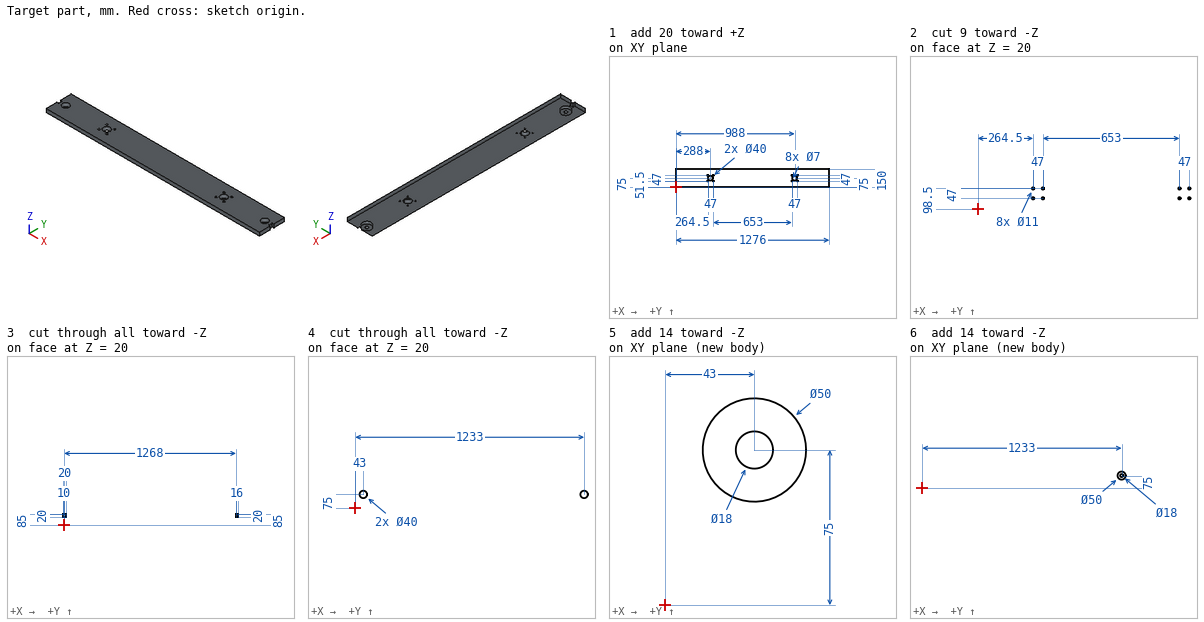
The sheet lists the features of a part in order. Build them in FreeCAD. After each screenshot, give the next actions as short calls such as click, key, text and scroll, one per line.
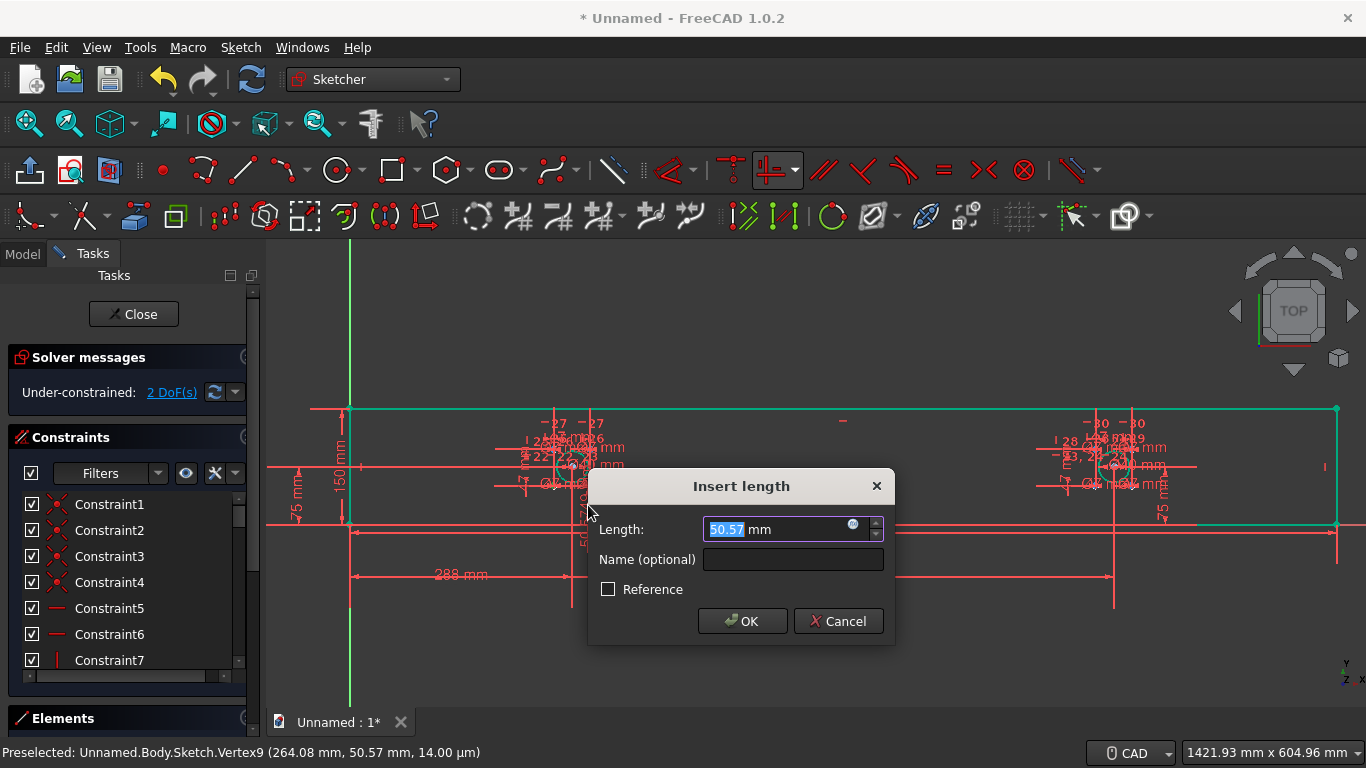
text(51.5)
key(Return)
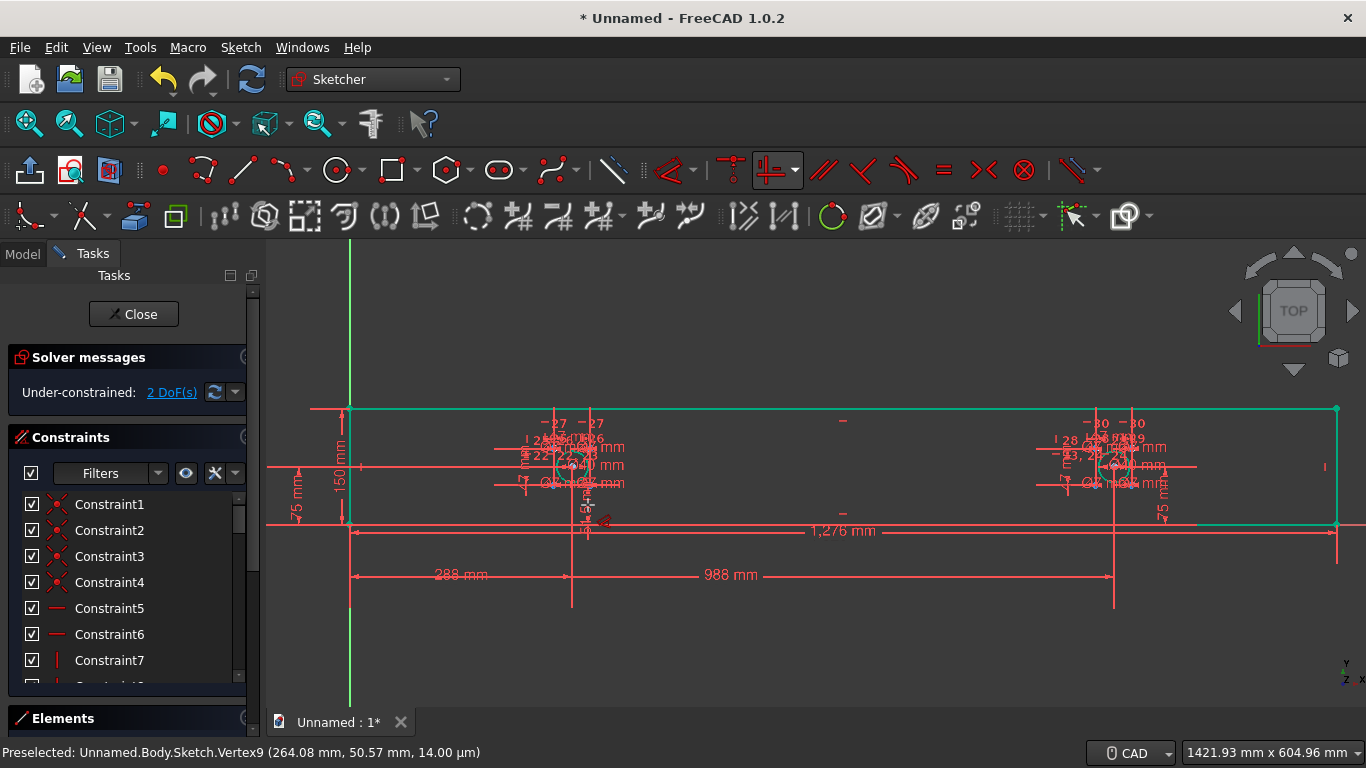
click(590, 485)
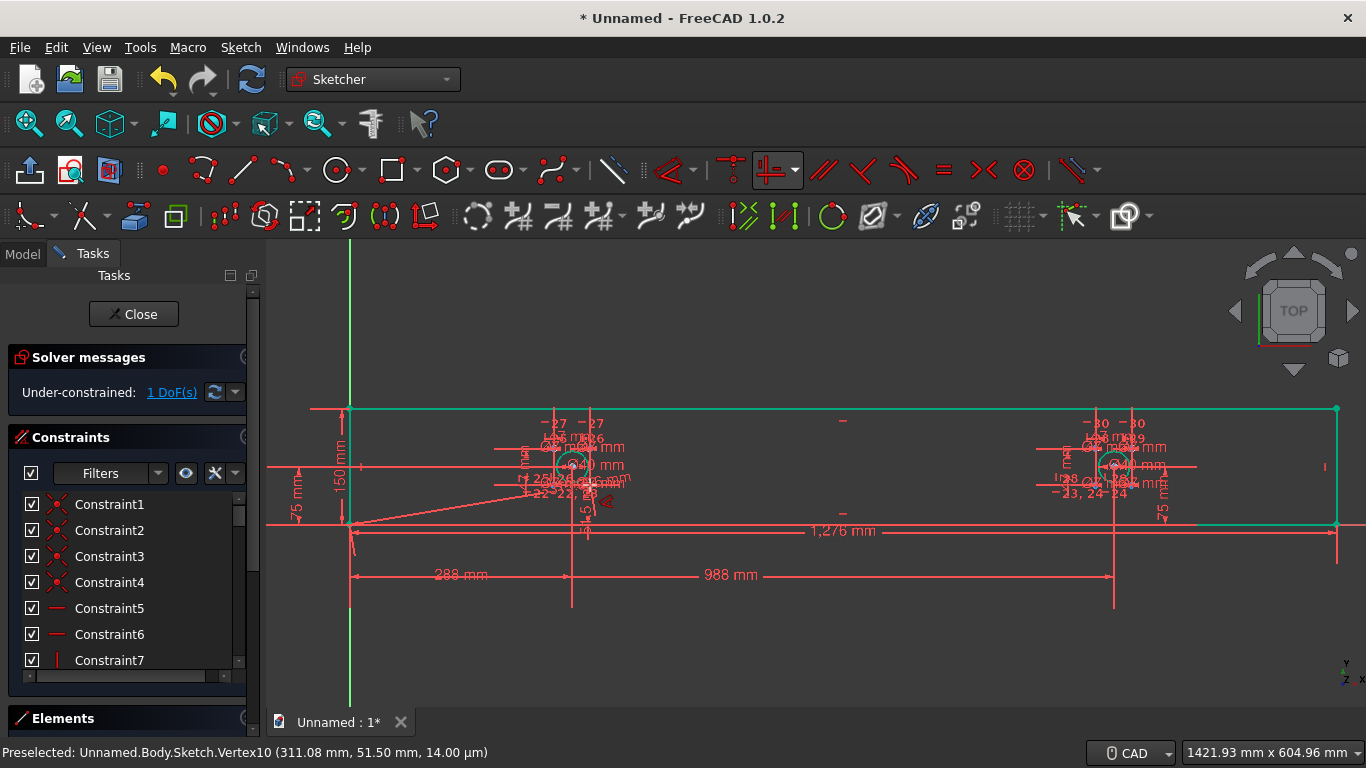
click(1096, 485)
click(843, 451)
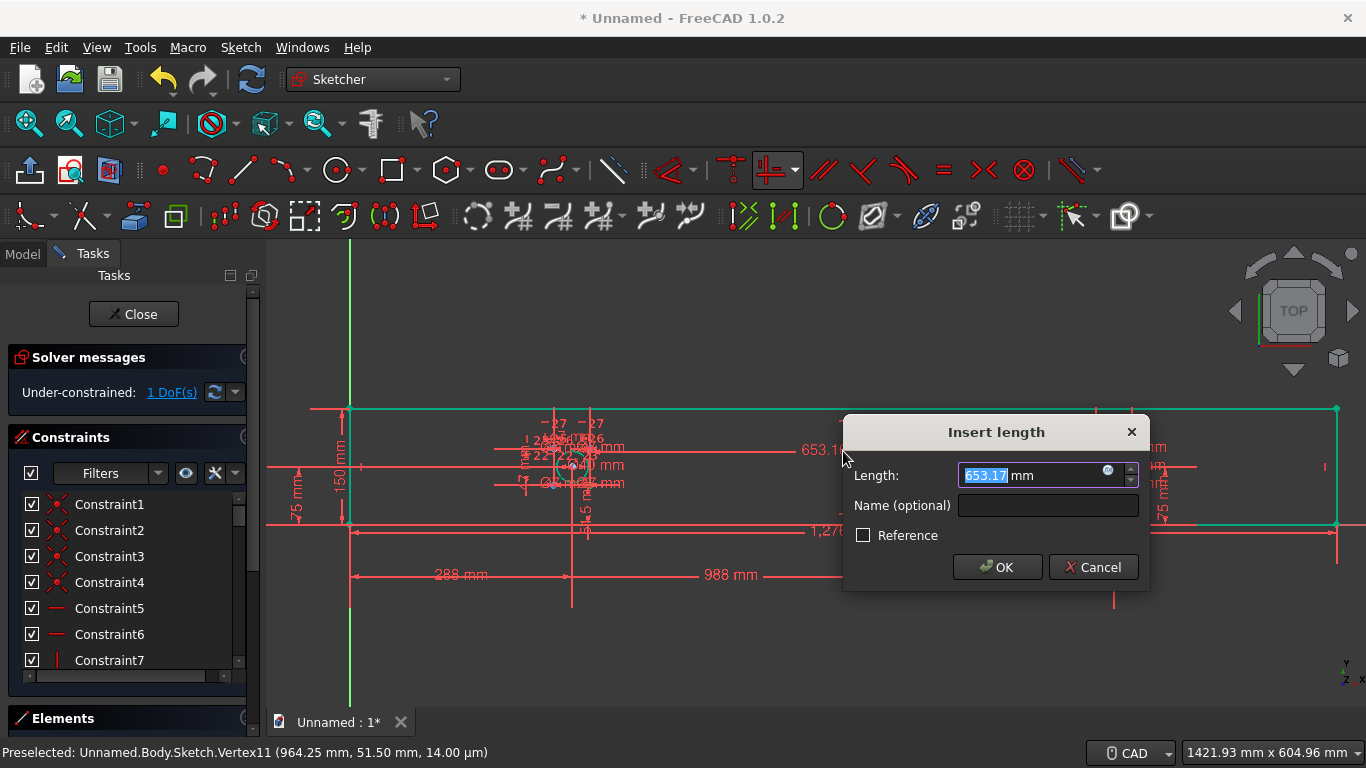
text(653)
key(Return)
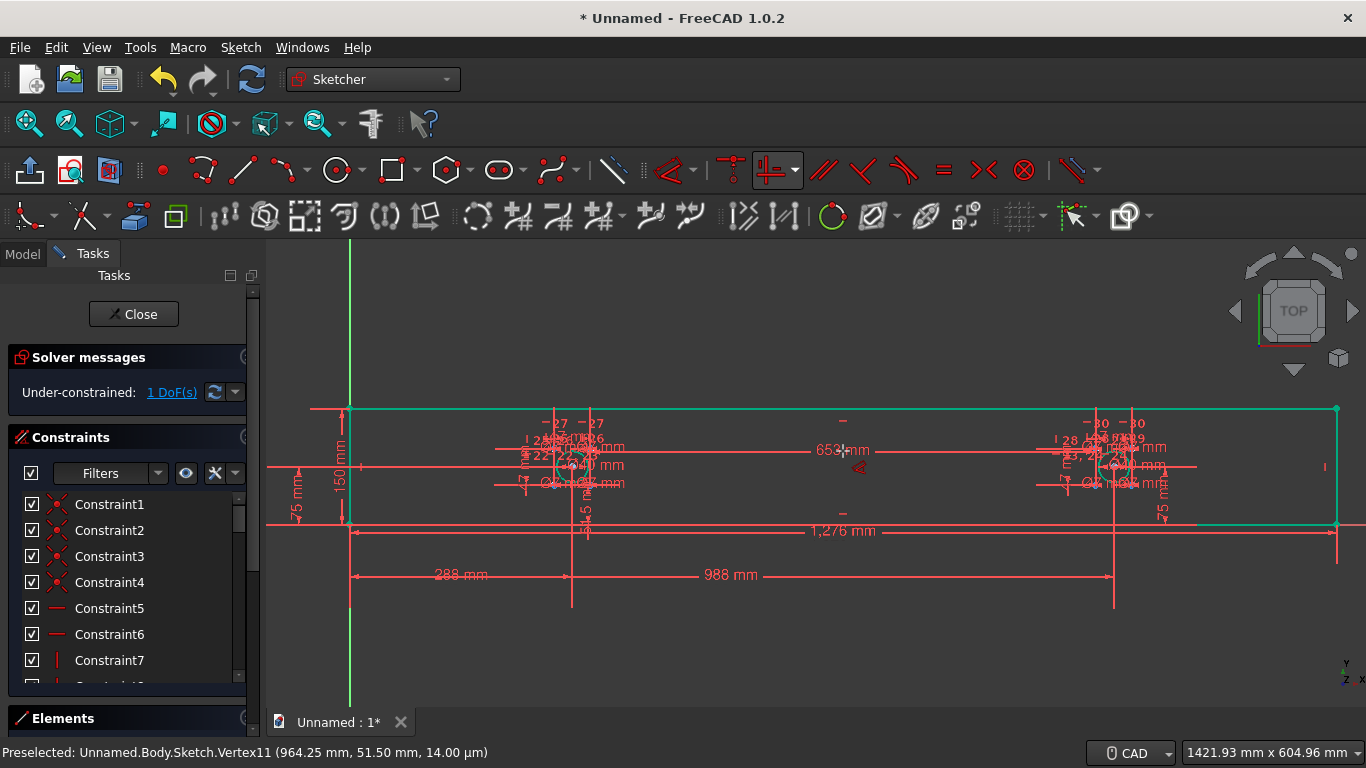
click(554, 485)
click(380, 559)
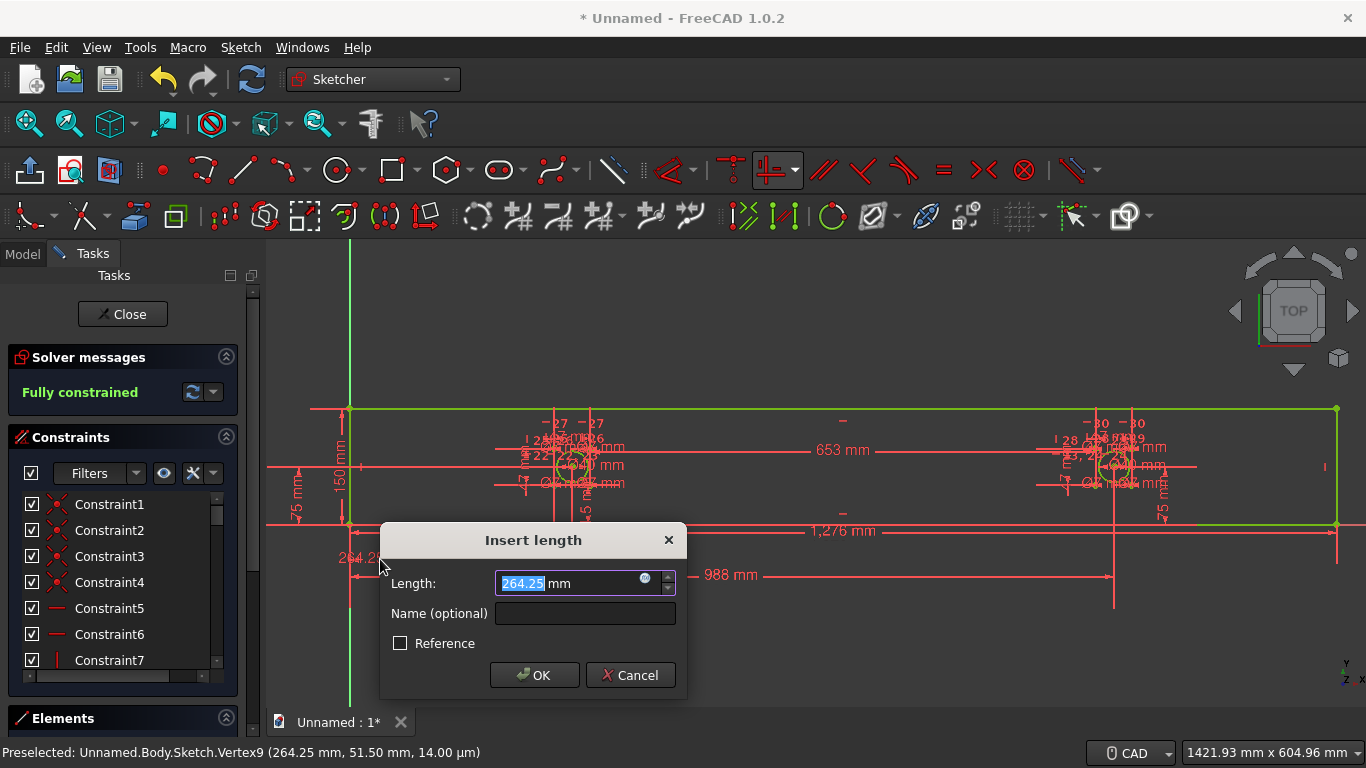
text(264.5)
key(Return)
key(Escape)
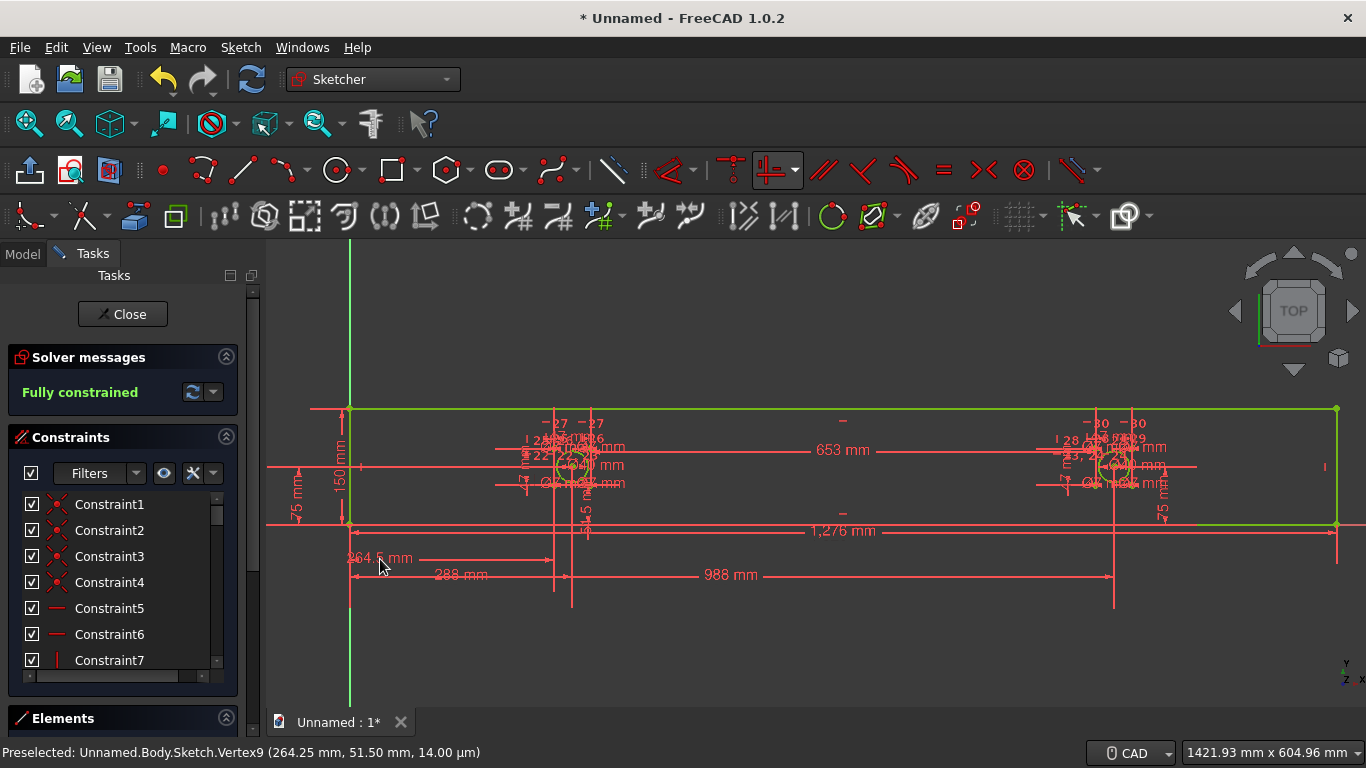
click(123, 314)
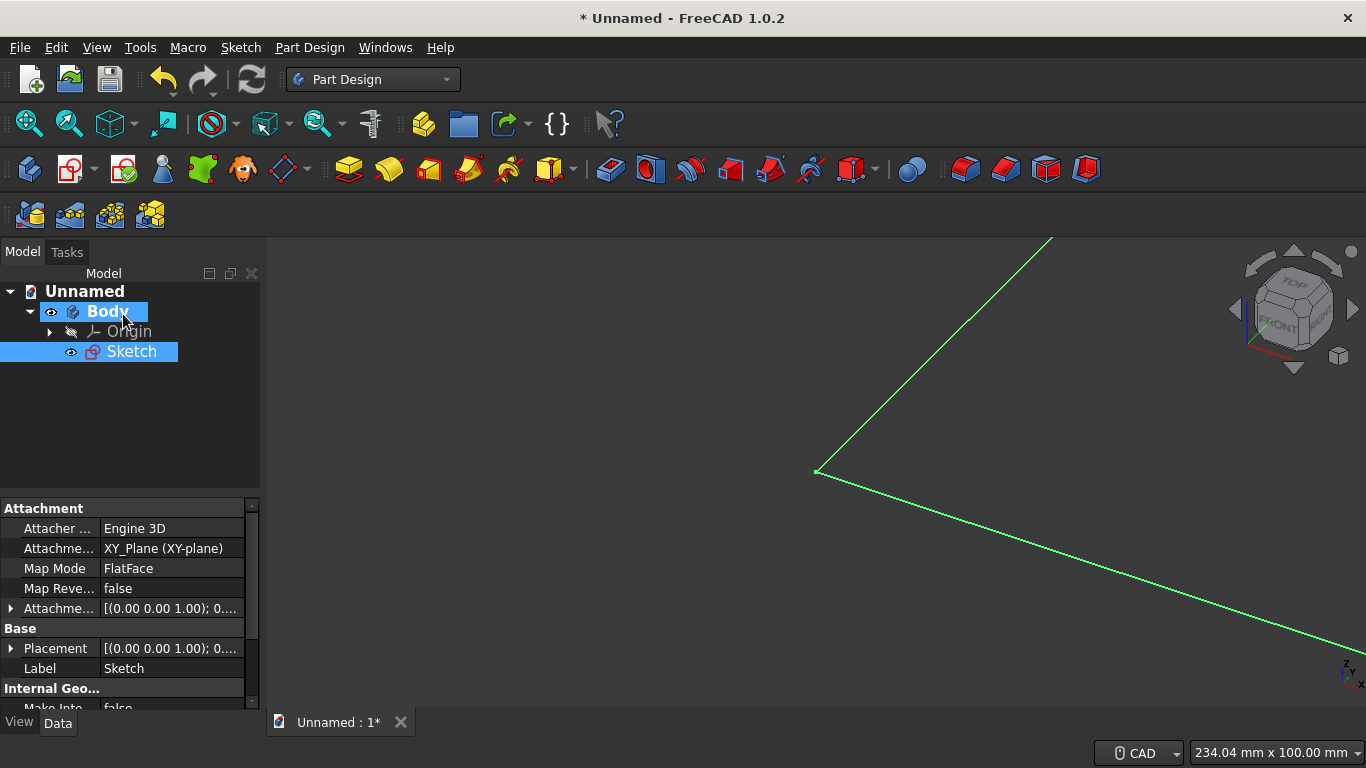
click(350, 170)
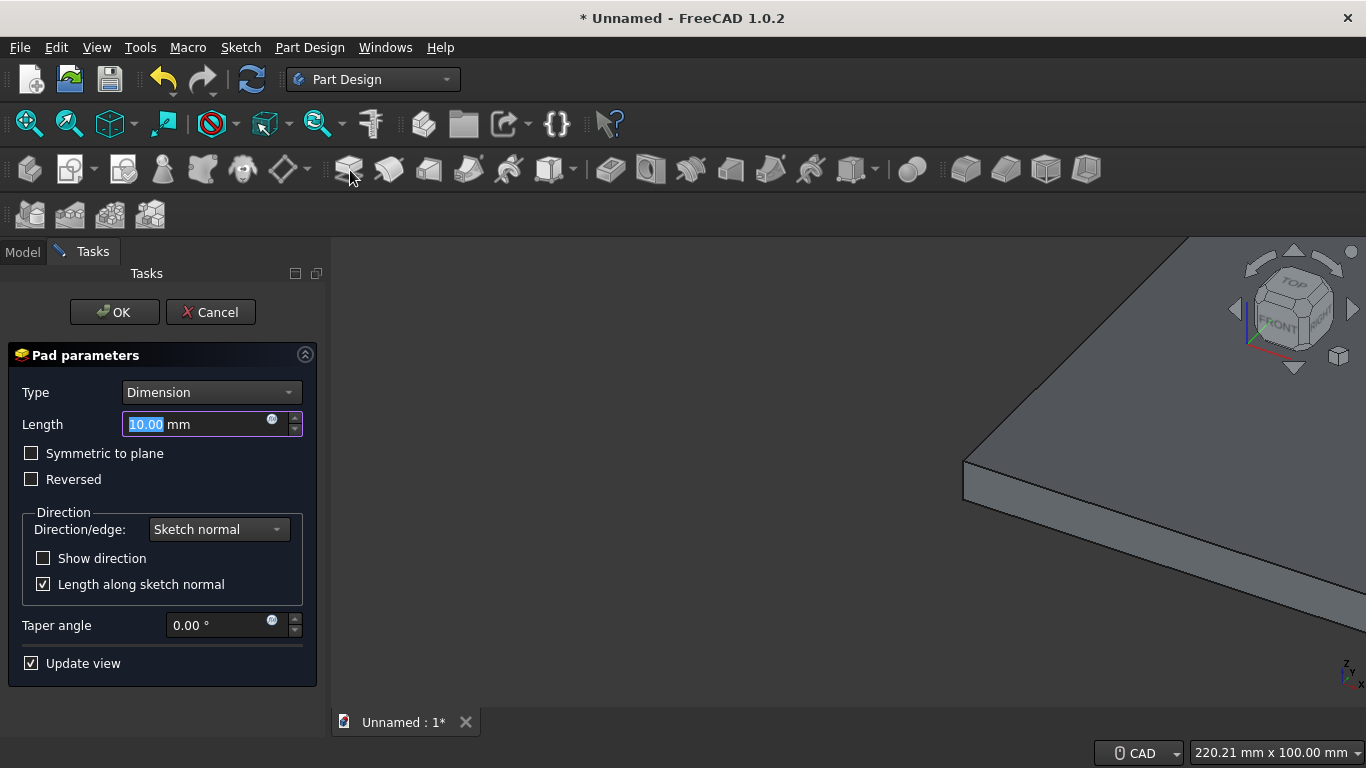
text(20)
key(Tab)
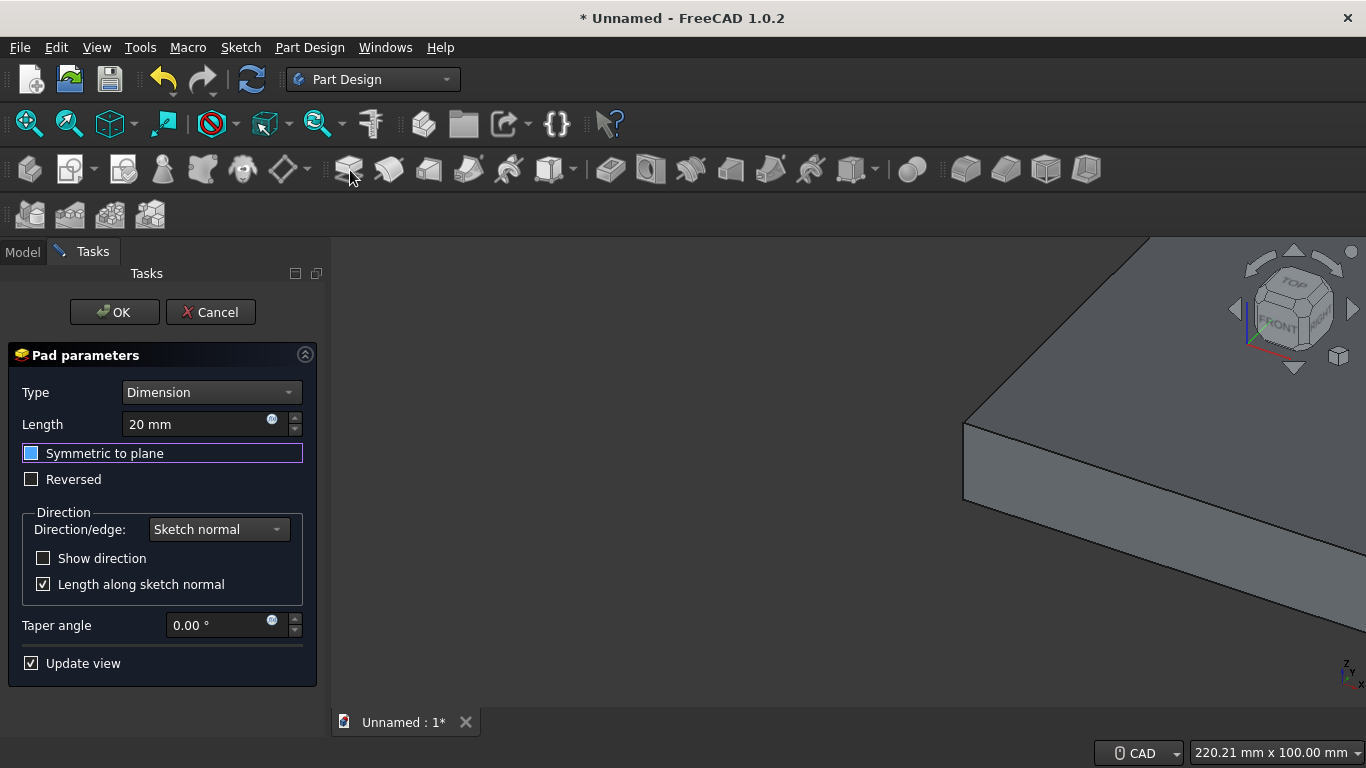
click(115, 312)